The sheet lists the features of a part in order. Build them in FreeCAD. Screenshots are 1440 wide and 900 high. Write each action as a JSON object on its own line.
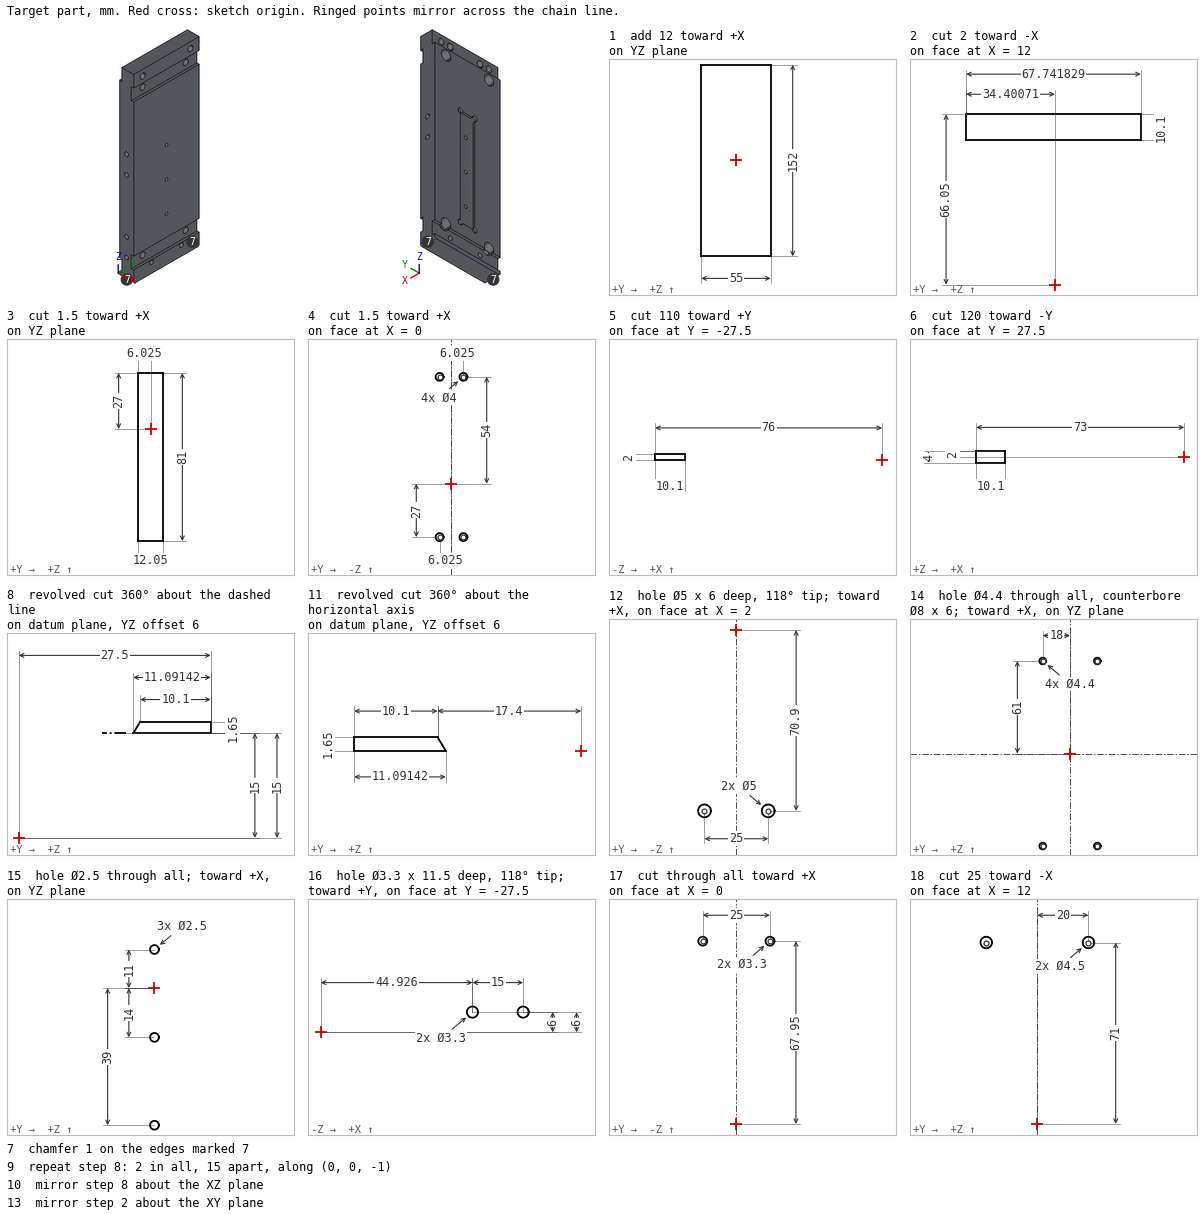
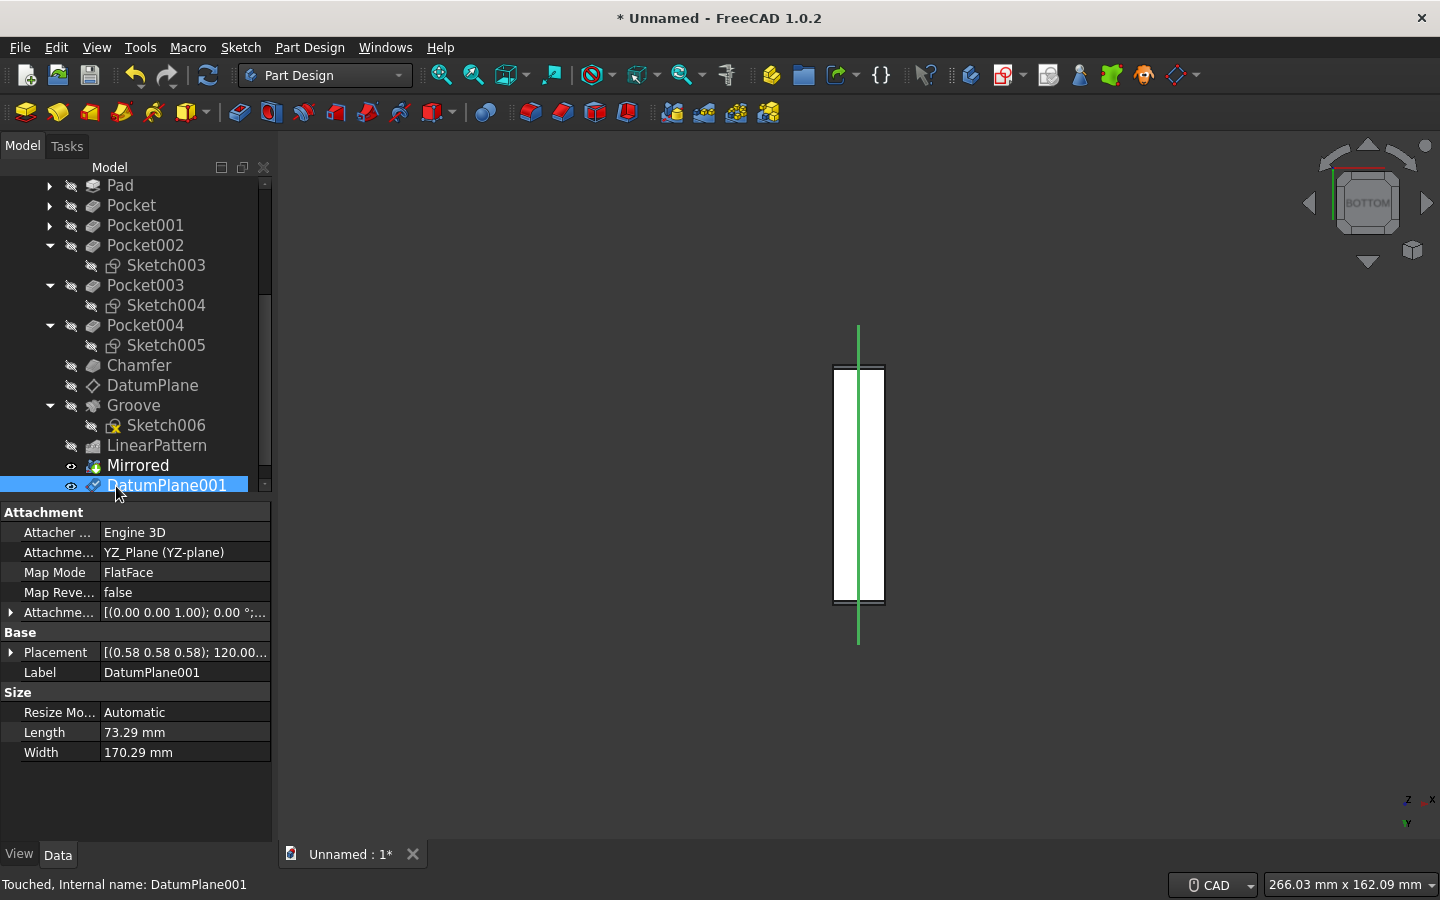
{"action": "left_click", "coordinate": [1004, 76]}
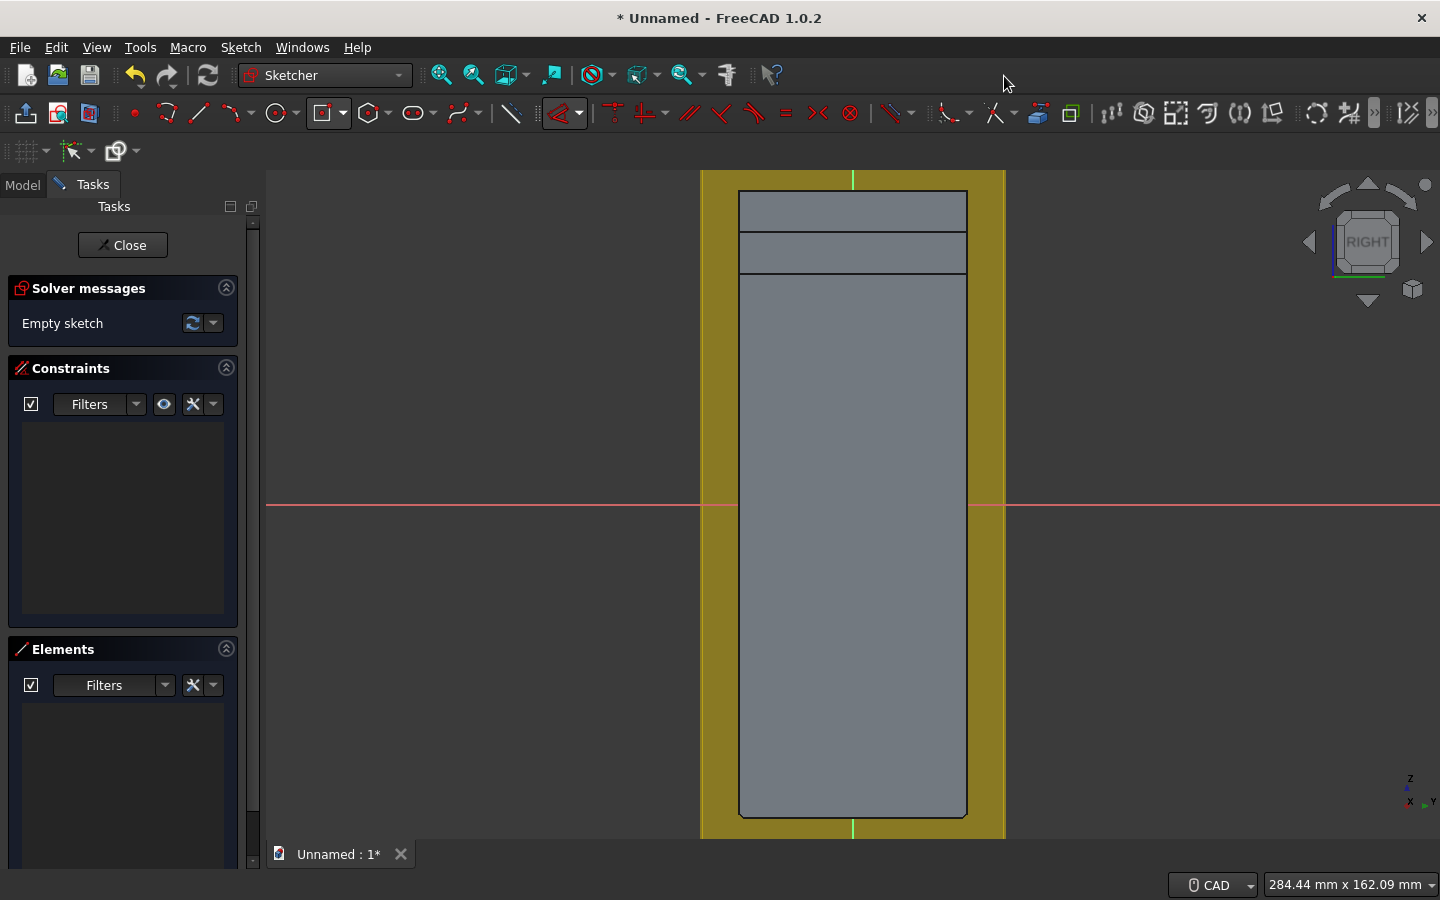
{"action": "left_click", "coordinate": [90, 114]}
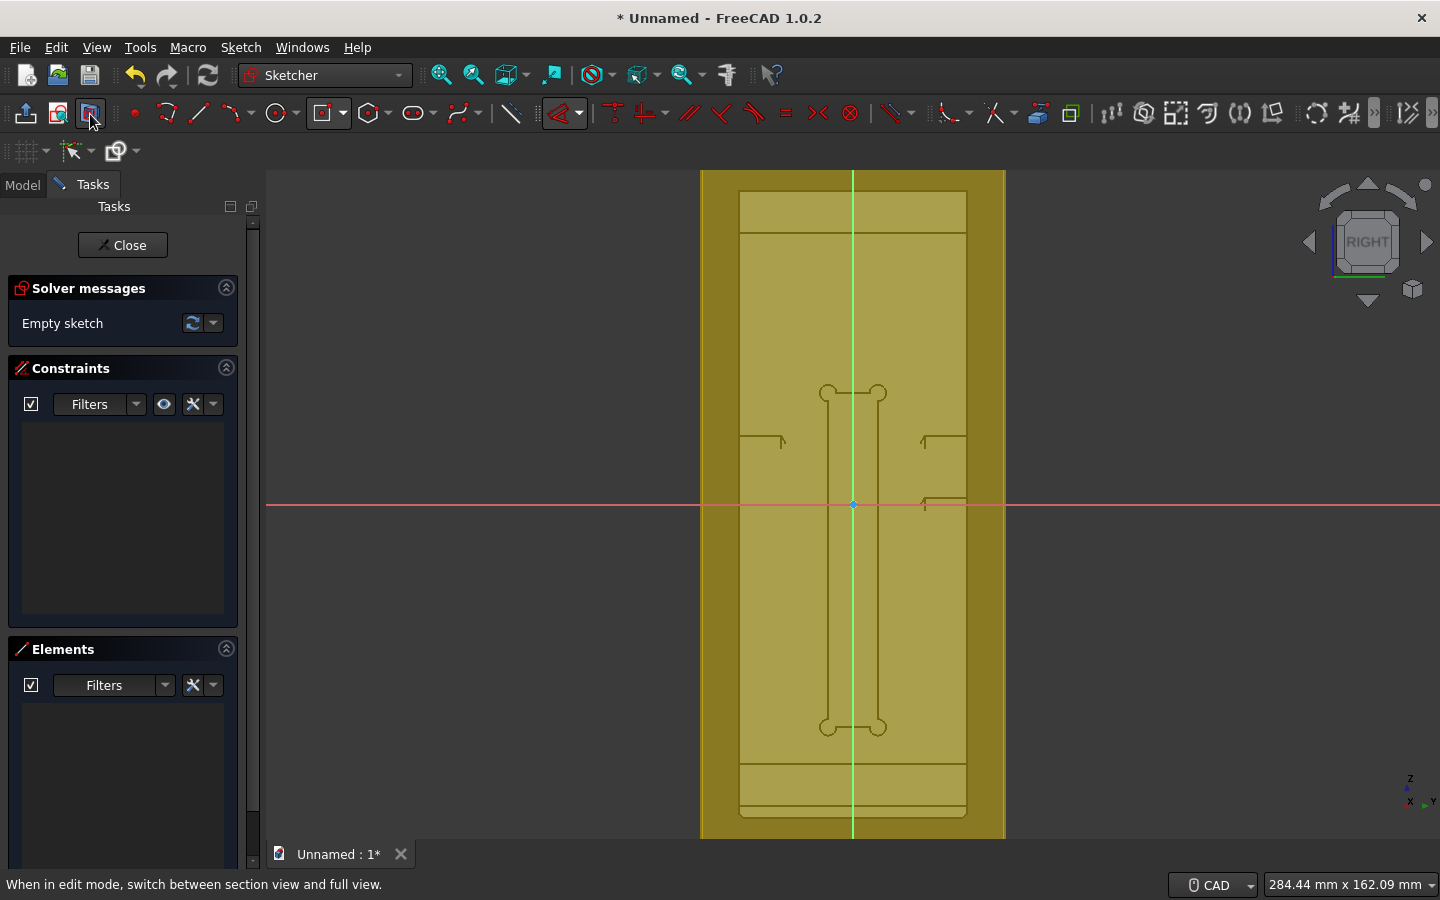
{"action": "scroll", "coordinate": [799, 500], "scroll_direction": "up", "scroll_amount": 9}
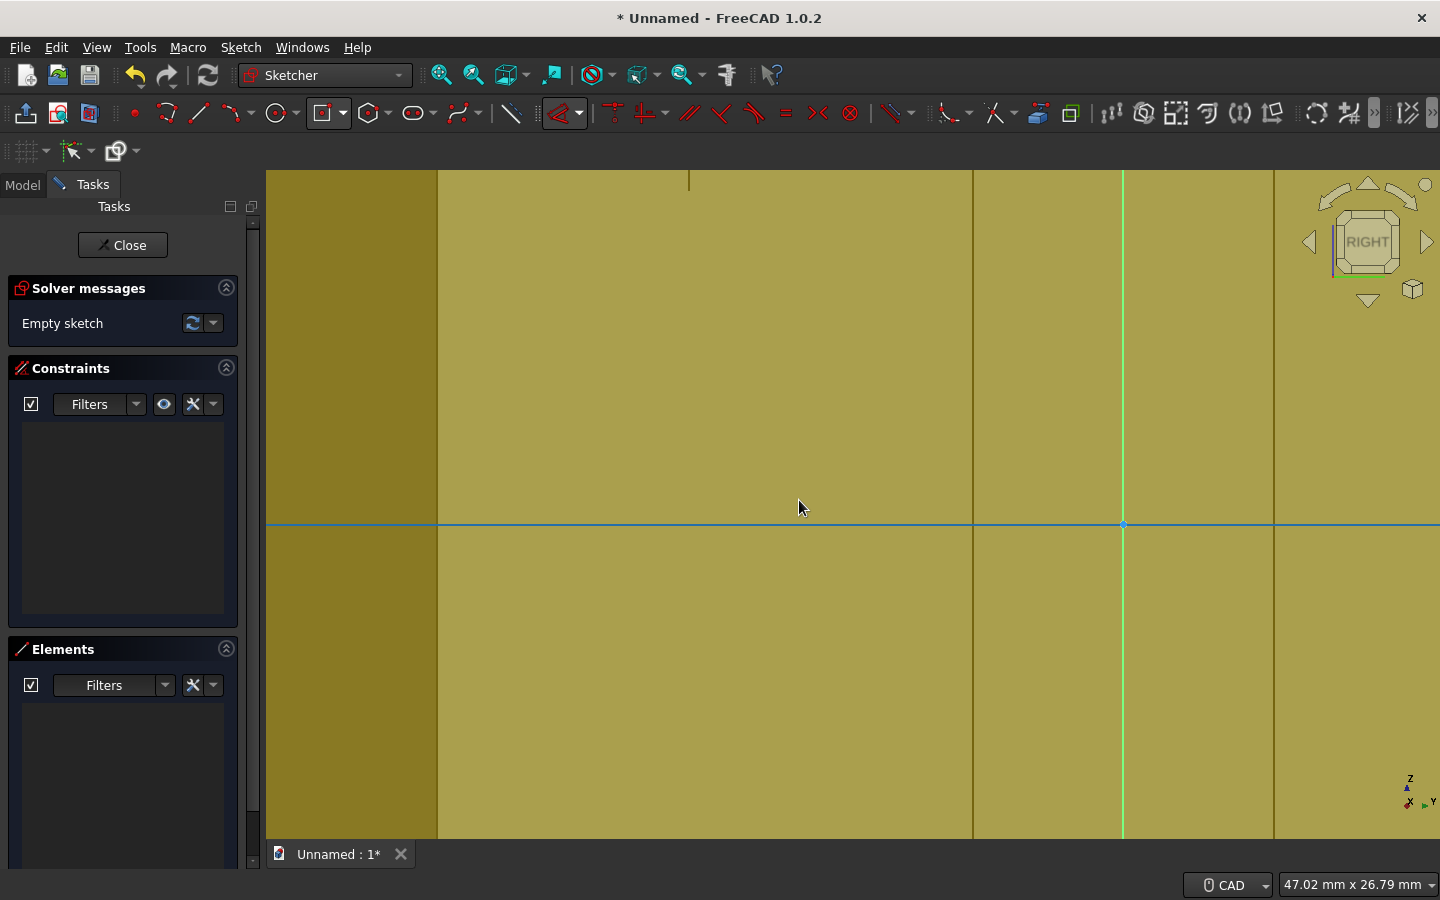
{"action": "left_click", "coordinate": [168, 114]}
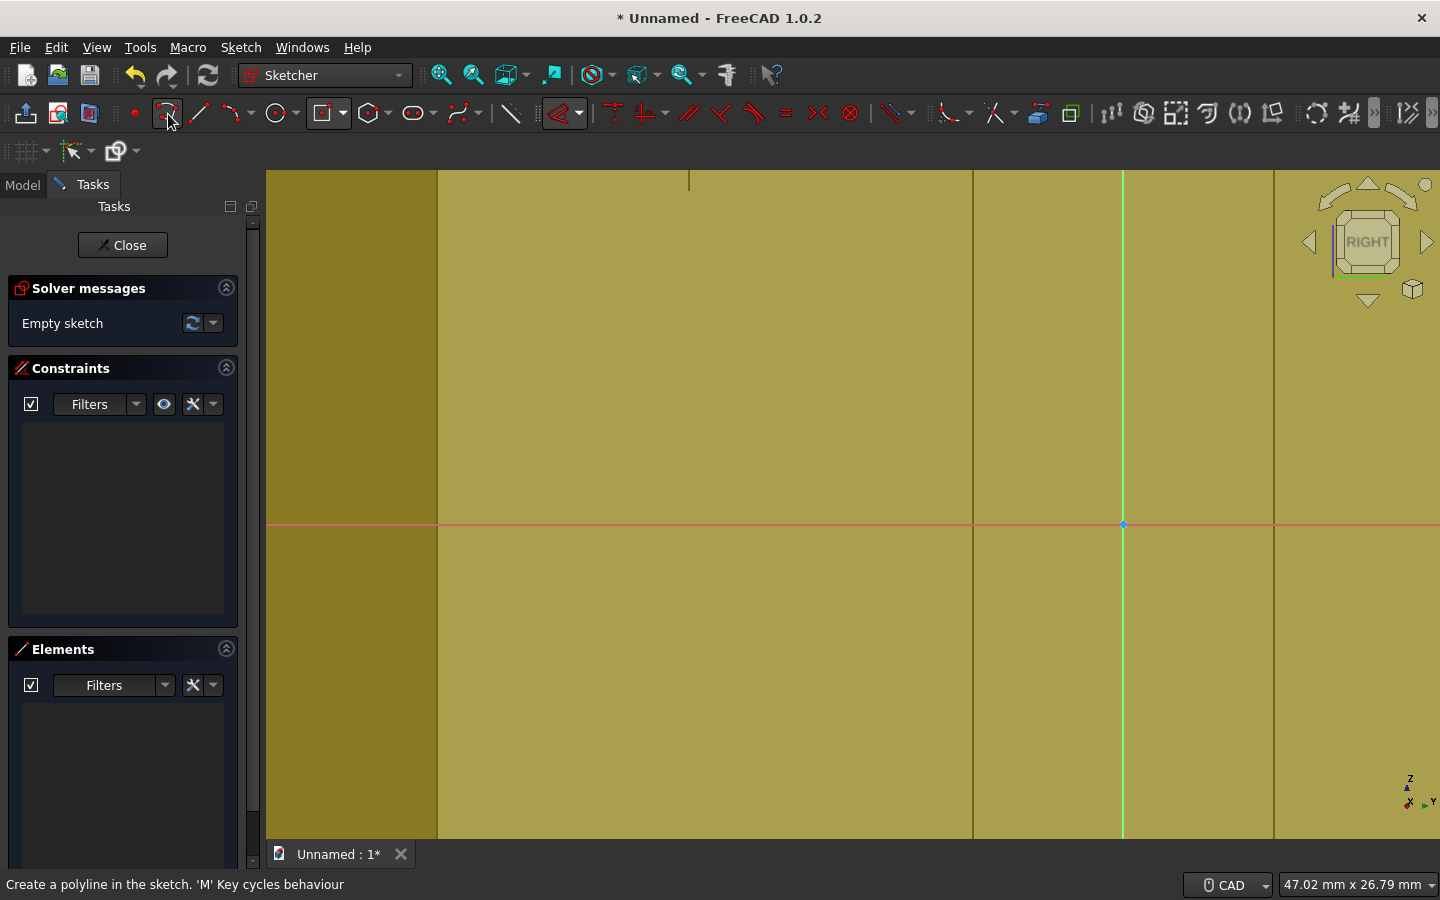
{"action": "left_click", "coordinate": [714, 525]}
{"action": "left_click", "coordinate": [689, 484]}
{"action": "left_click", "coordinate": [437, 484]}
{"action": "left_click", "coordinate": [437, 516]}
{"action": "left_click", "coordinate": [714, 525]}
{"action": "key", "text": "Escape"}
{"action": "key", "text": "Escape"}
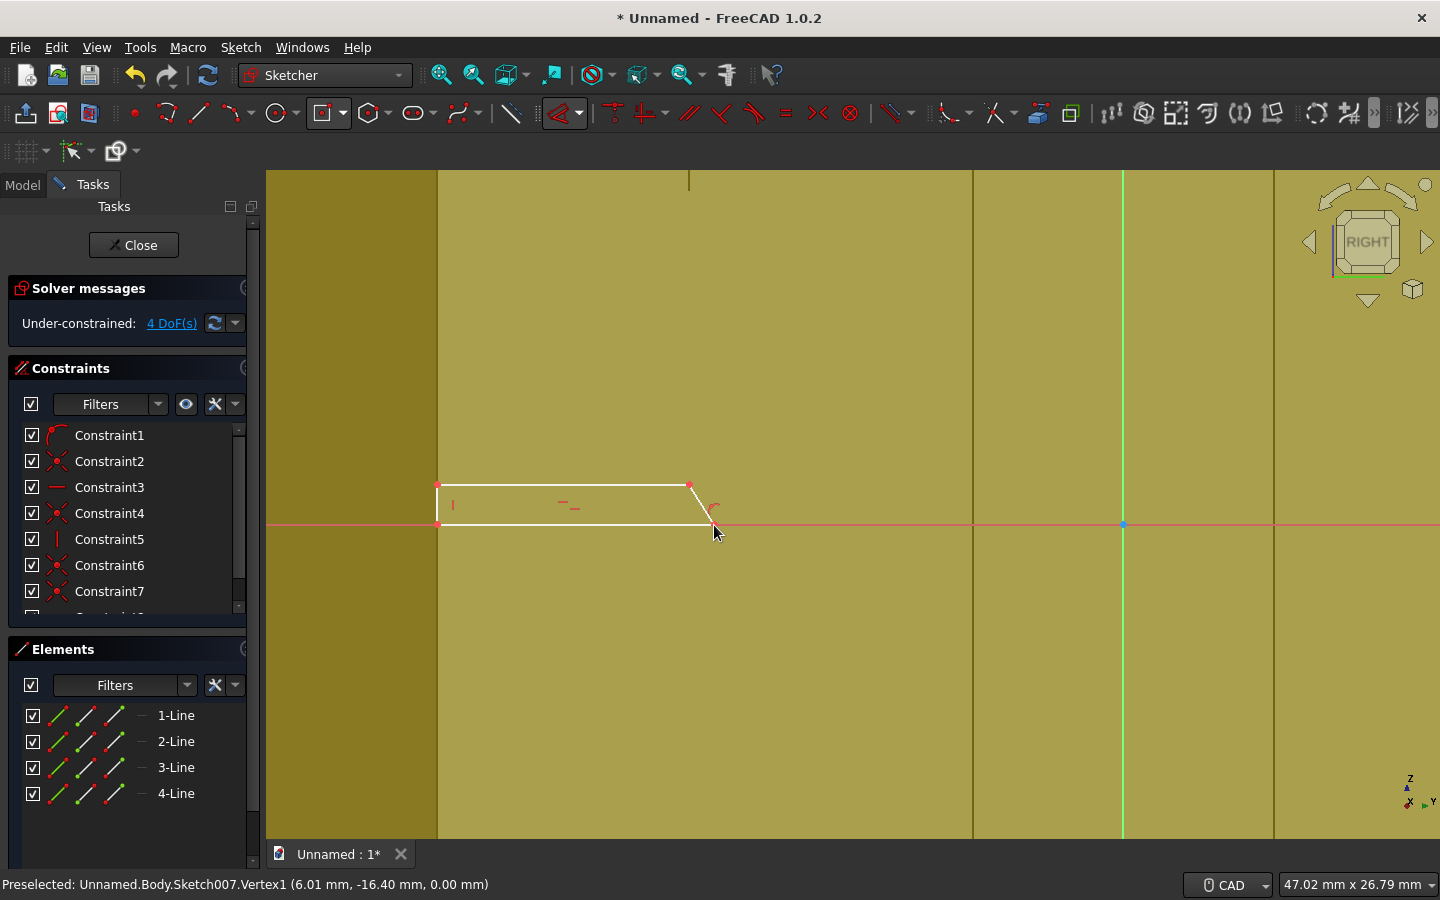
{"action": "left_click", "coordinate": [613, 485]}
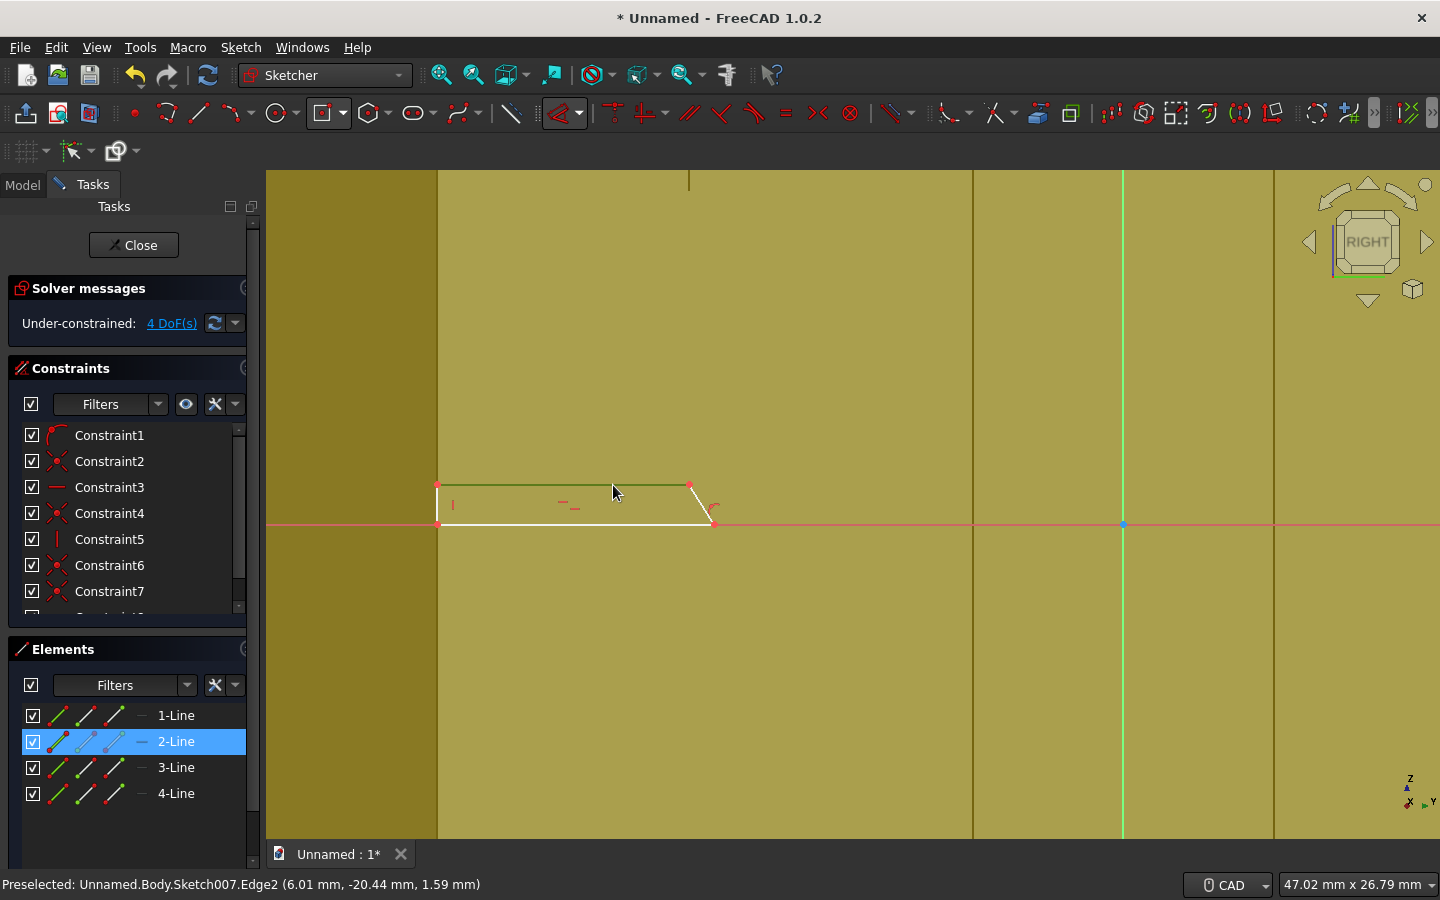
{"action": "key", "text": "l"}